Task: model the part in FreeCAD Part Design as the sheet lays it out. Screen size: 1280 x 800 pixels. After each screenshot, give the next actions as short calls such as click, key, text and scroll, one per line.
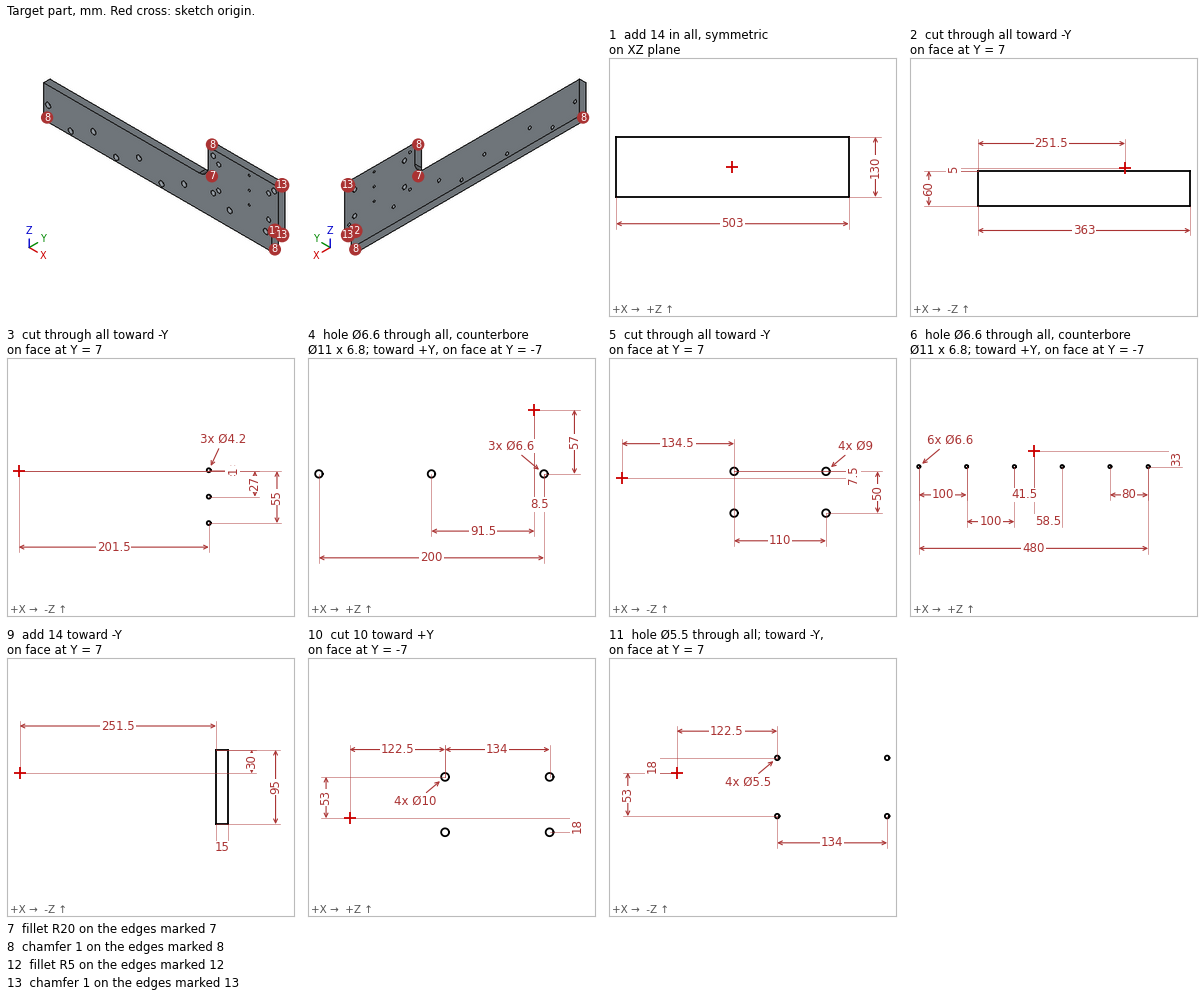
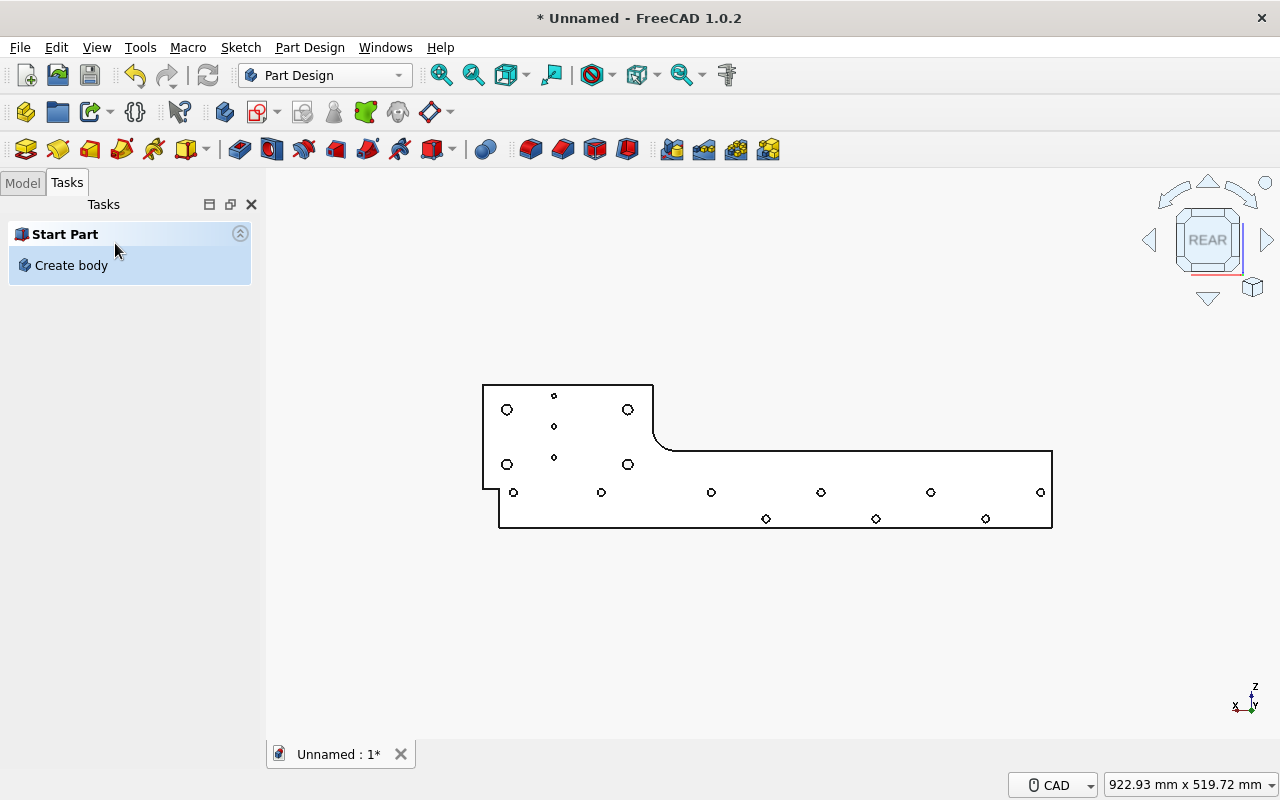
click(605, 435)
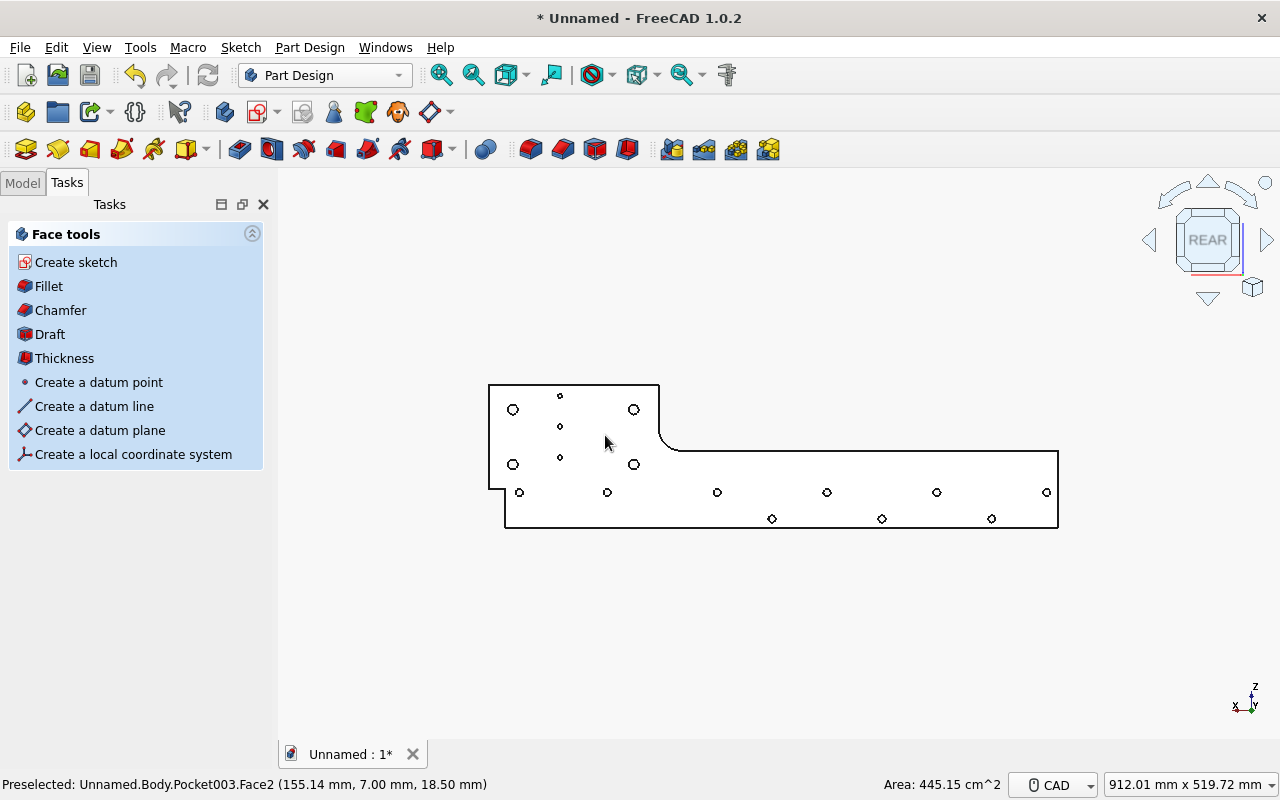
click(258, 112)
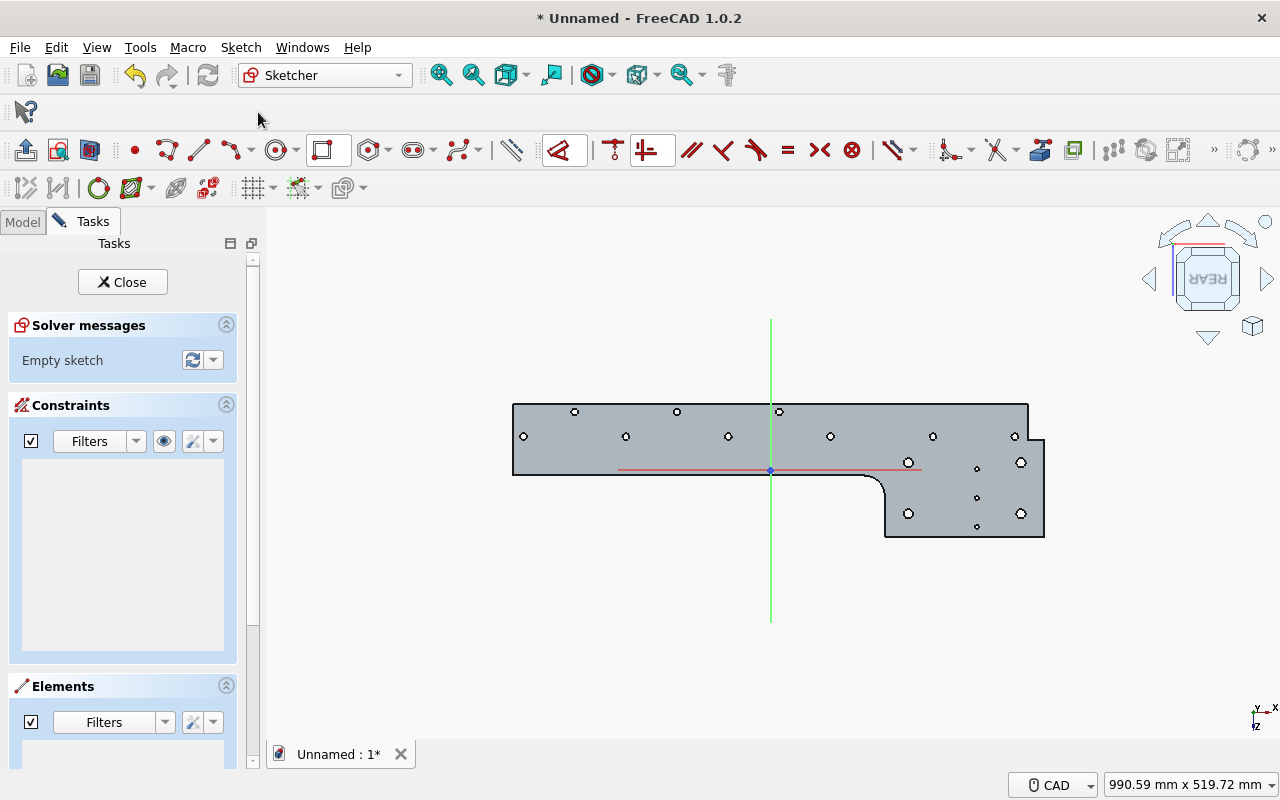
scroll(1066, 501, up, 4)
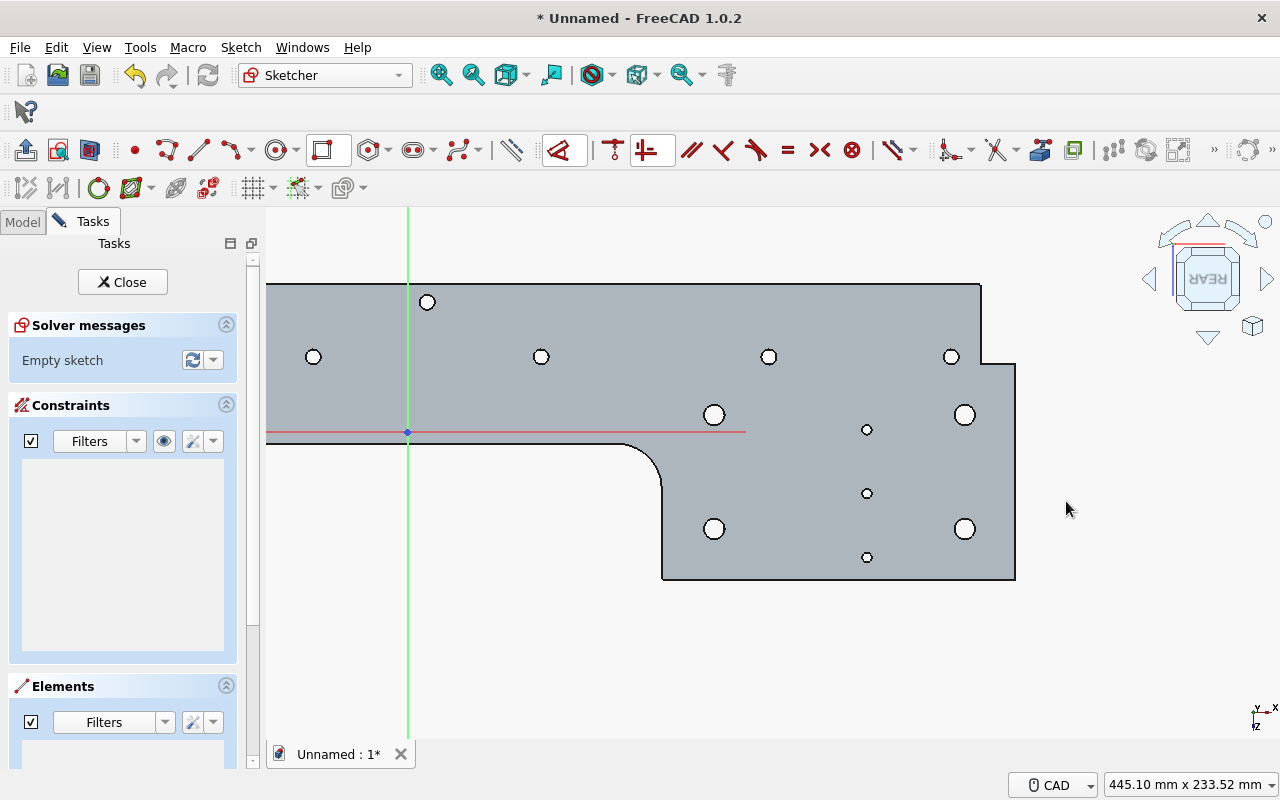
key(g)
key(c)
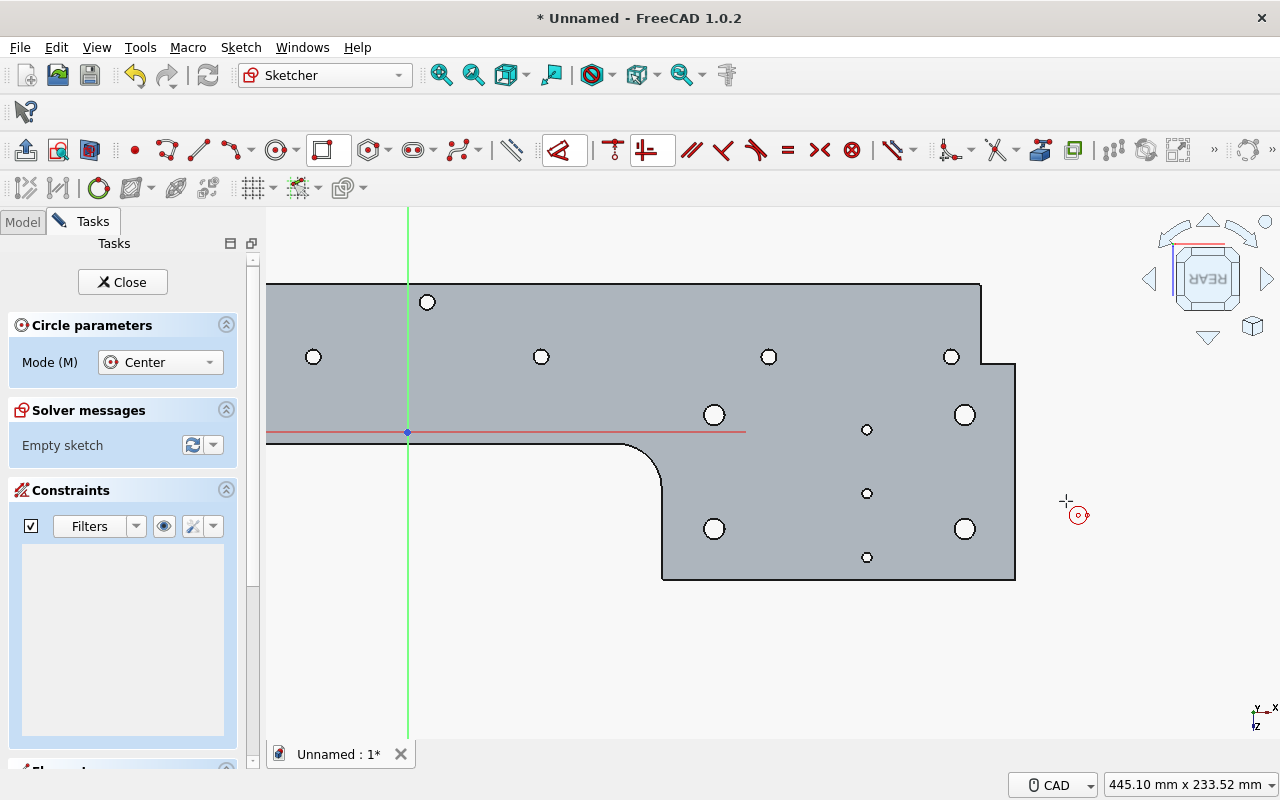
scroll(687, 391, up, 7)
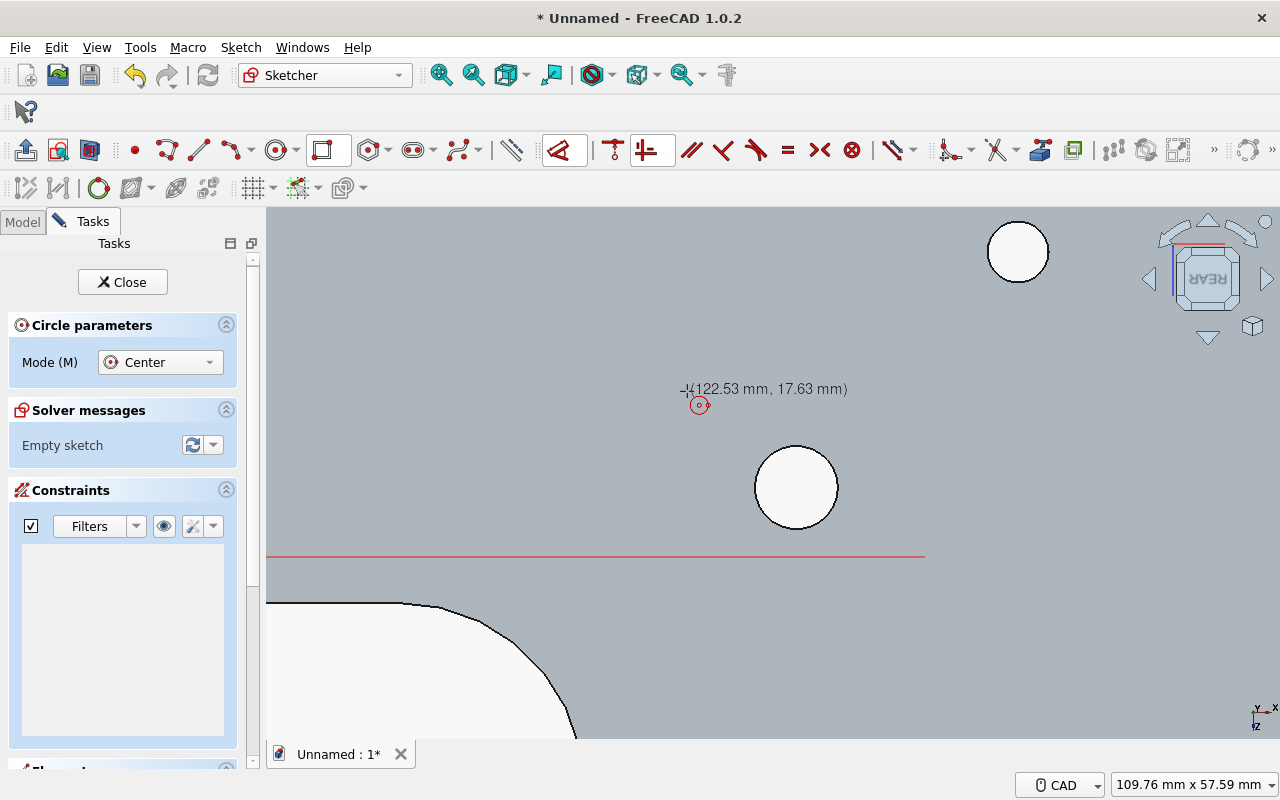
scroll(689, 393, down, 7)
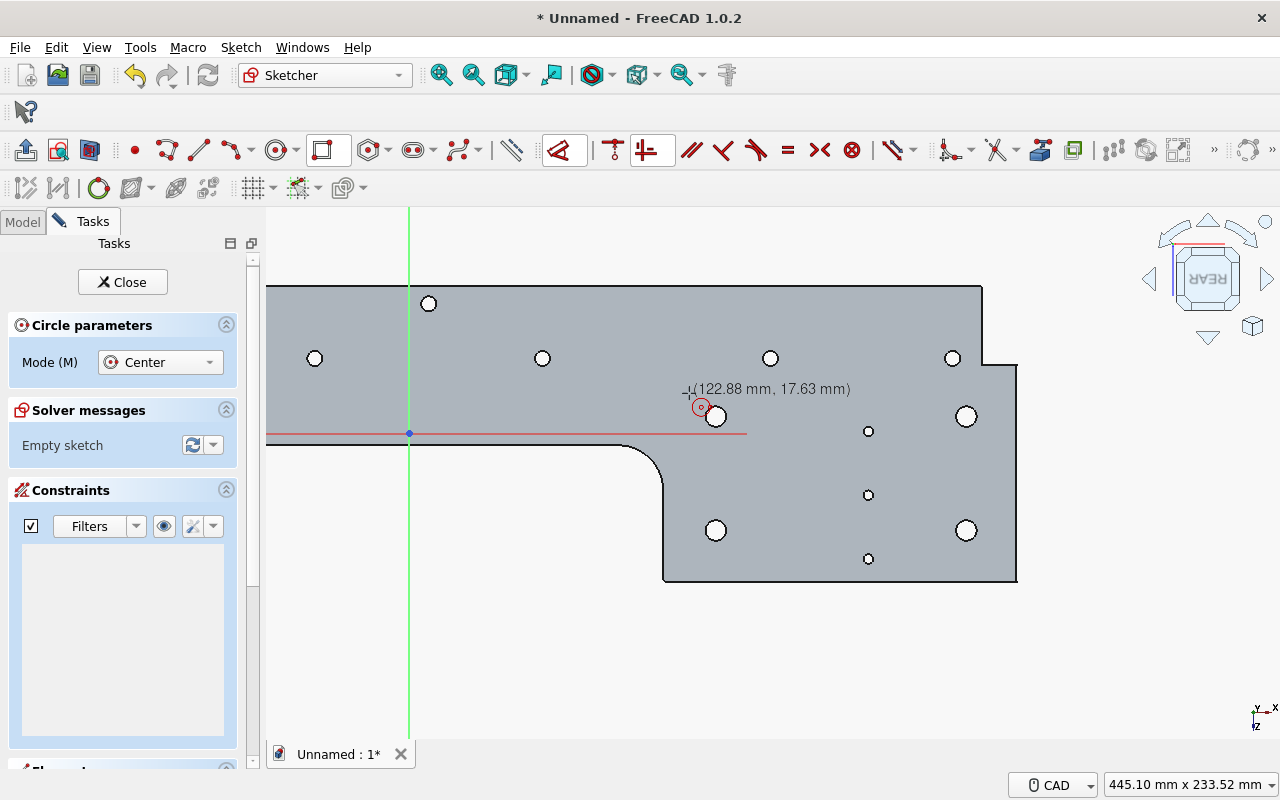
click(688, 393)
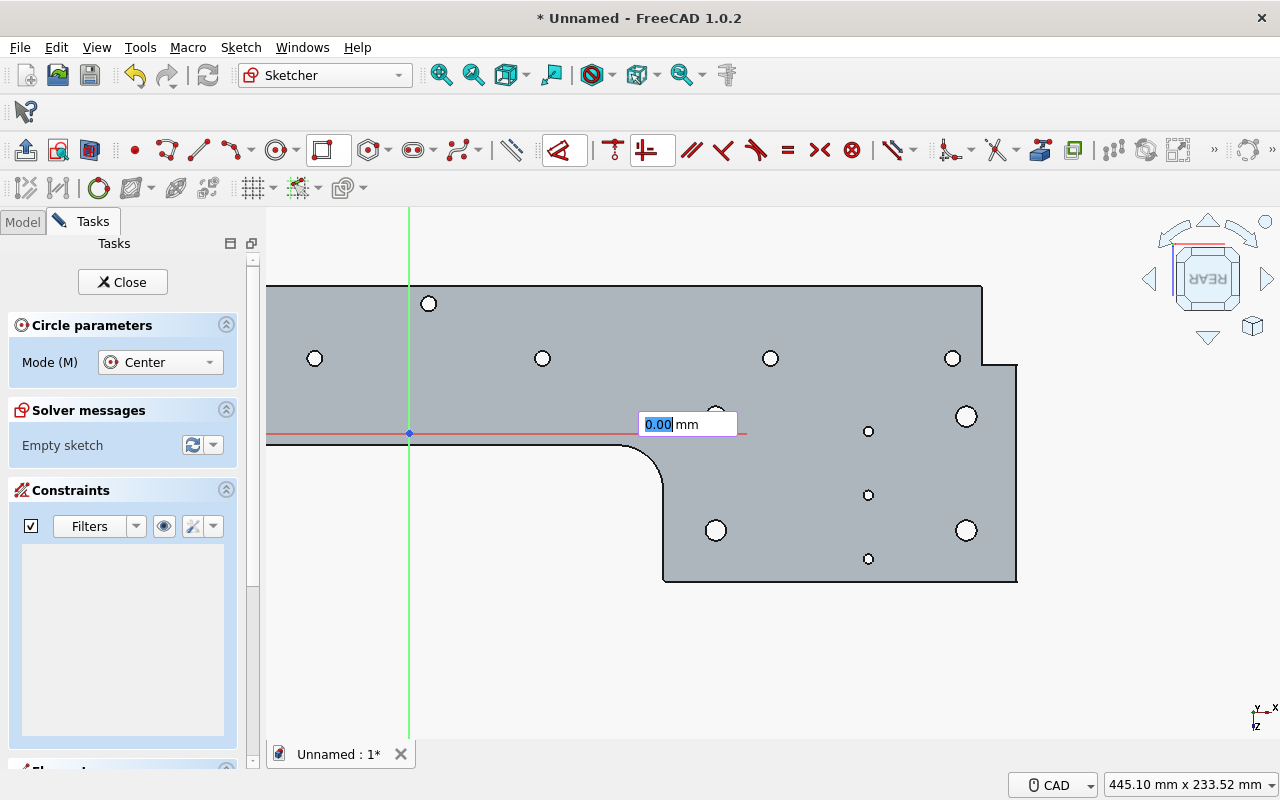
scroll(693, 388, up, 5)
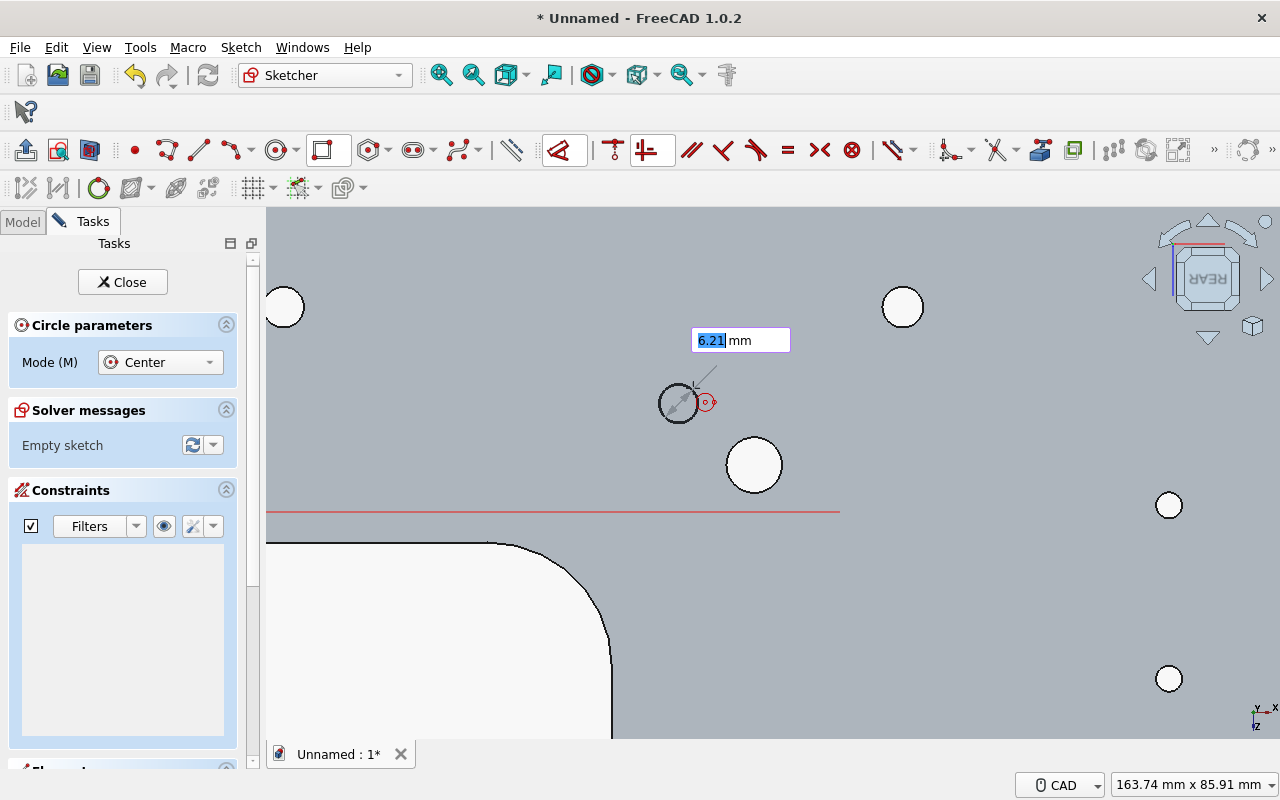
click(692, 388)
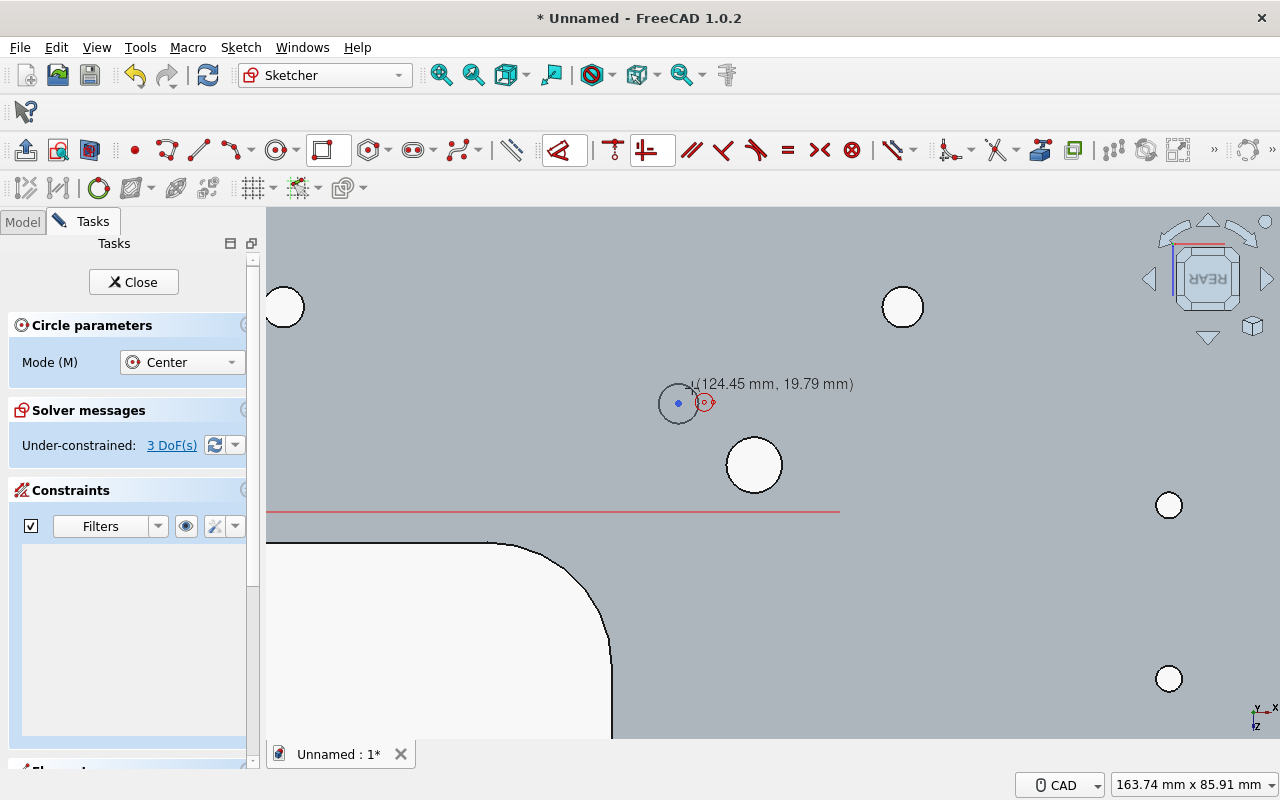
scroll(693, 387, down, 5)